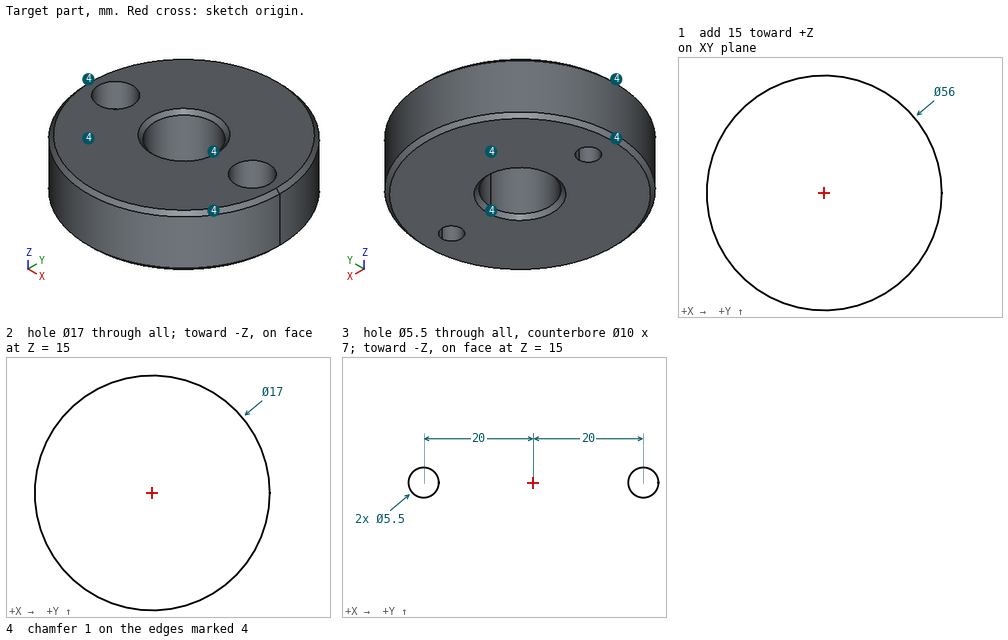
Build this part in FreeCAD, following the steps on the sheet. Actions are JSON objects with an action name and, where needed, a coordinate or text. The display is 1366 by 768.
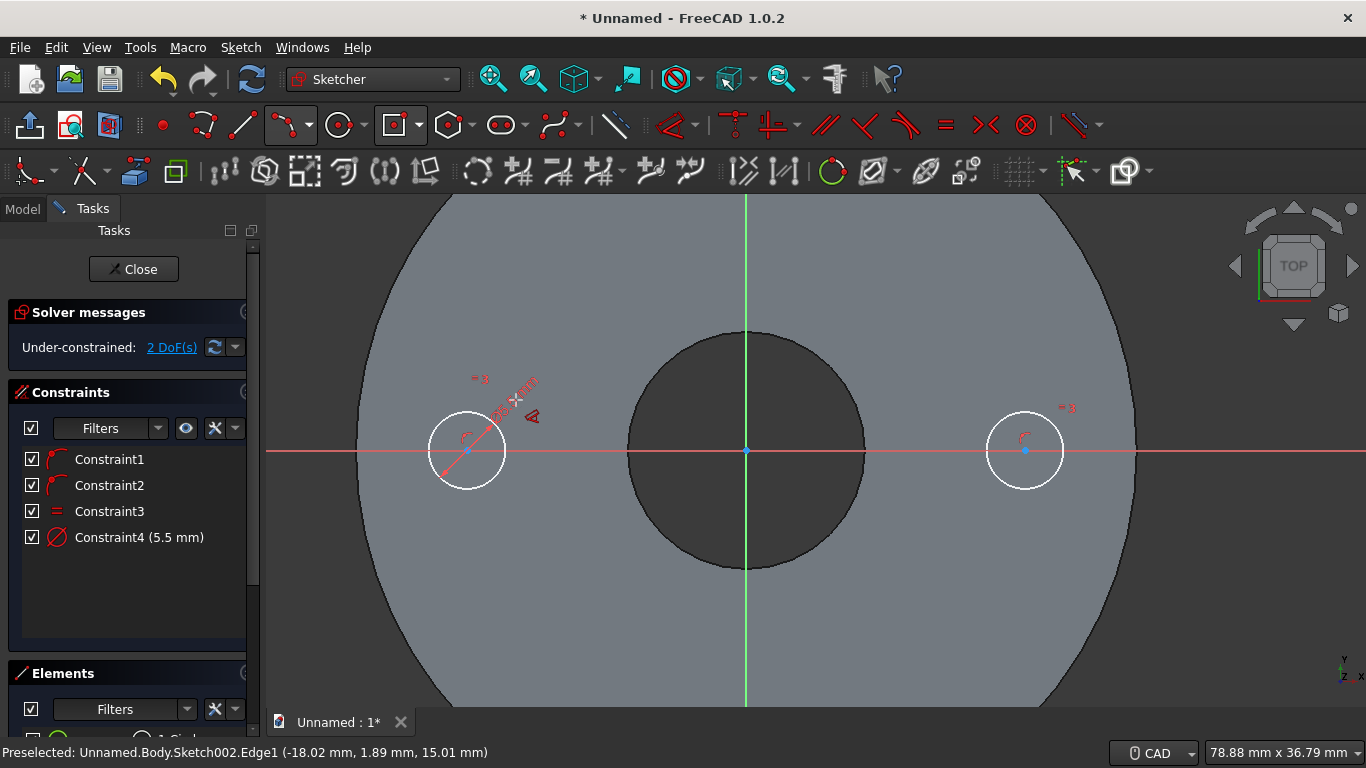
{"action": "left_click", "coordinate": [467, 450]}
{"action": "left_click", "coordinate": [607, 484]}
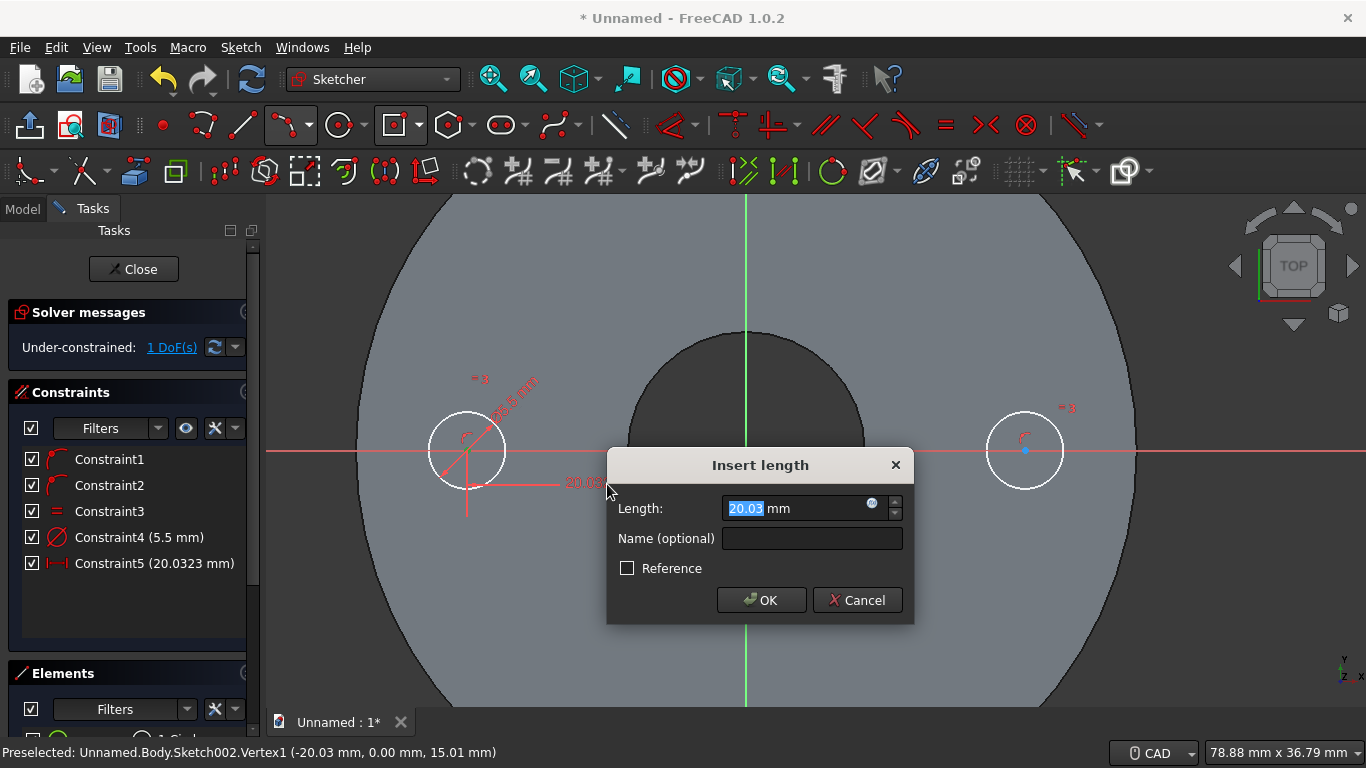
{"action": "type", "text": "20"}
{"action": "key", "text": "Return"}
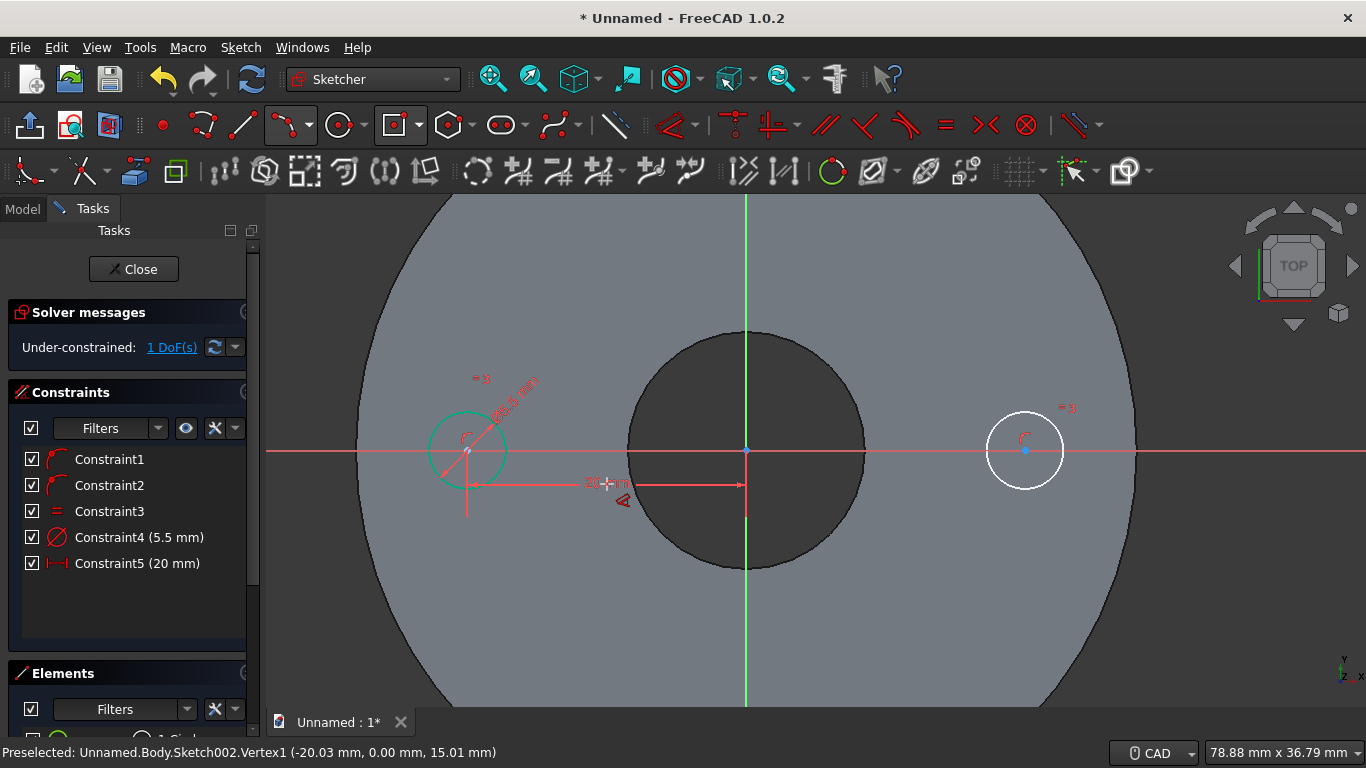
{"action": "left_click", "coordinate": [1025, 450]}
{"action": "left_click", "coordinate": [886, 484]}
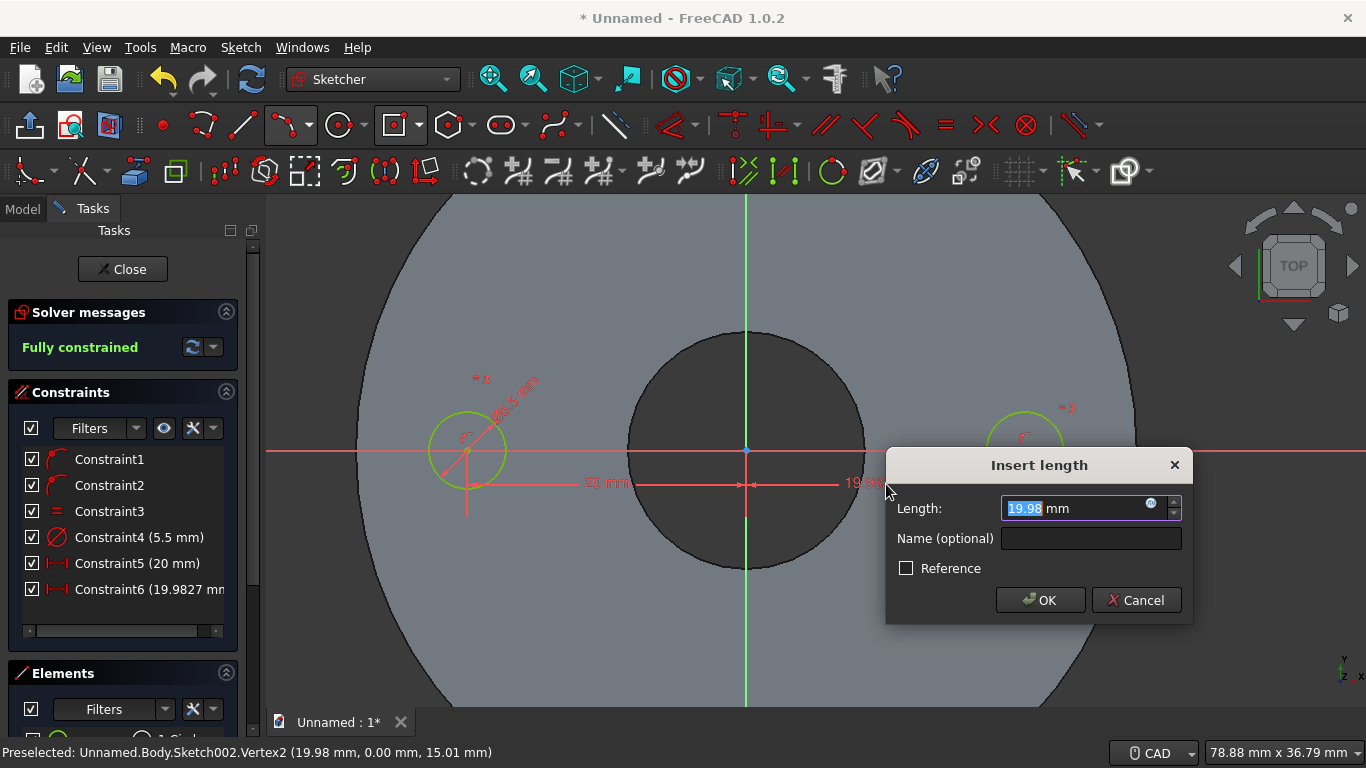
{"action": "type", "text": "20"}
{"action": "key", "text": "Return"}
{"action": "key", "text": "Escape"}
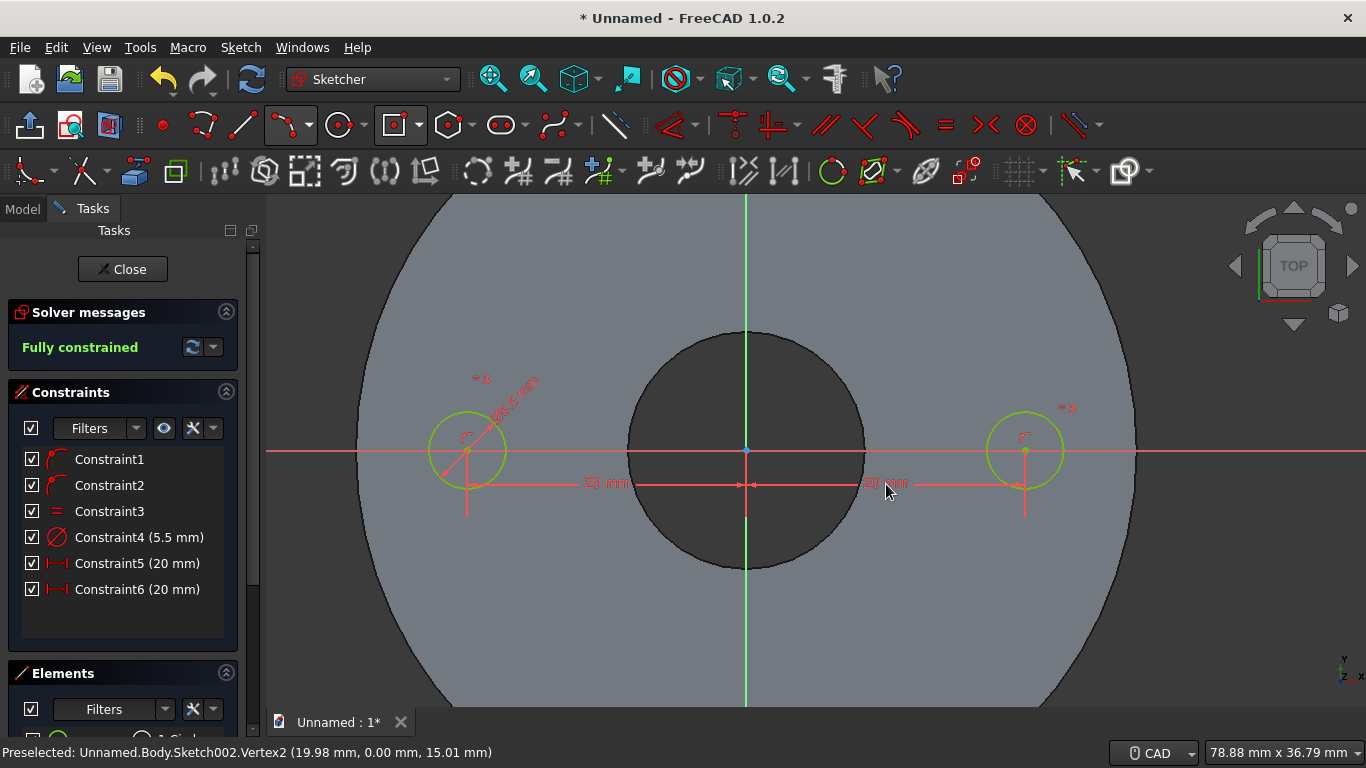
{"action": "left_click", "coordinate": [123, 269]}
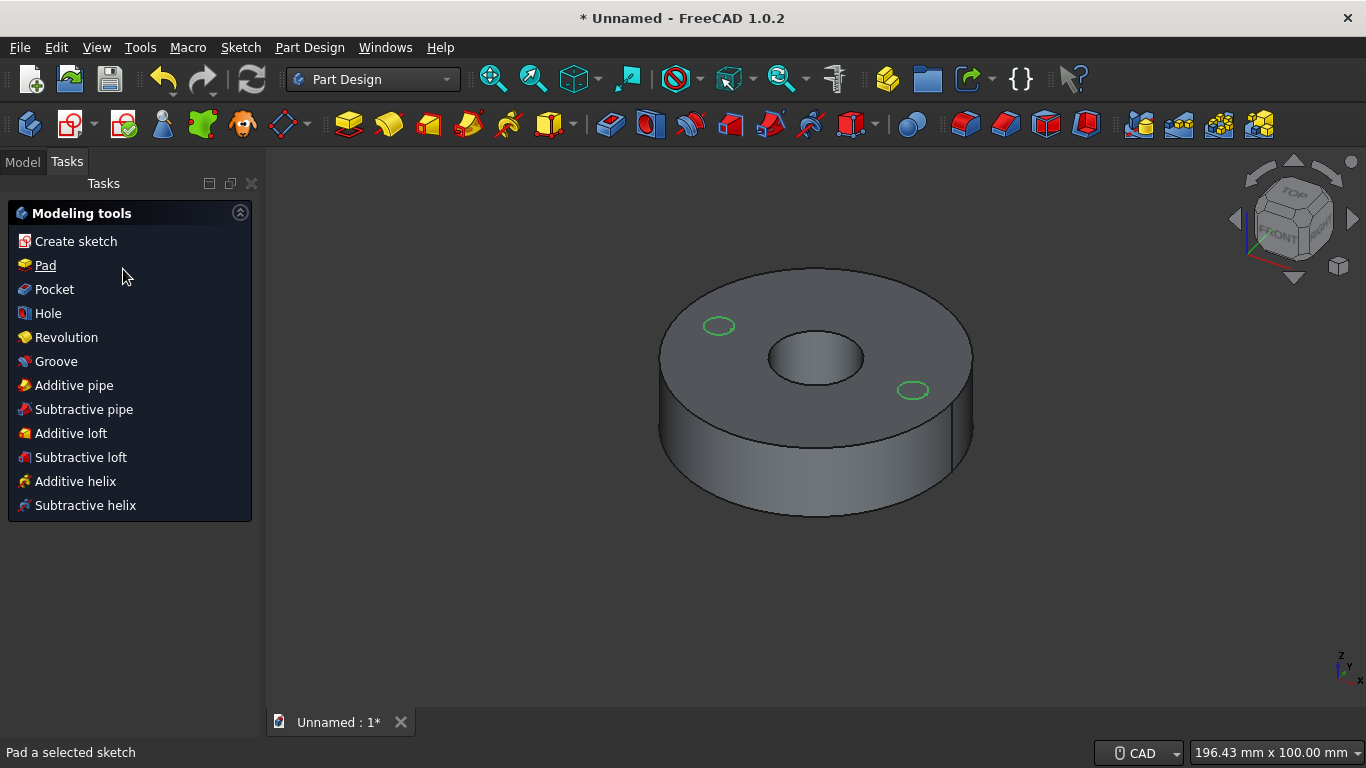
{"action": "left_click", "coordinate": [652, 124]}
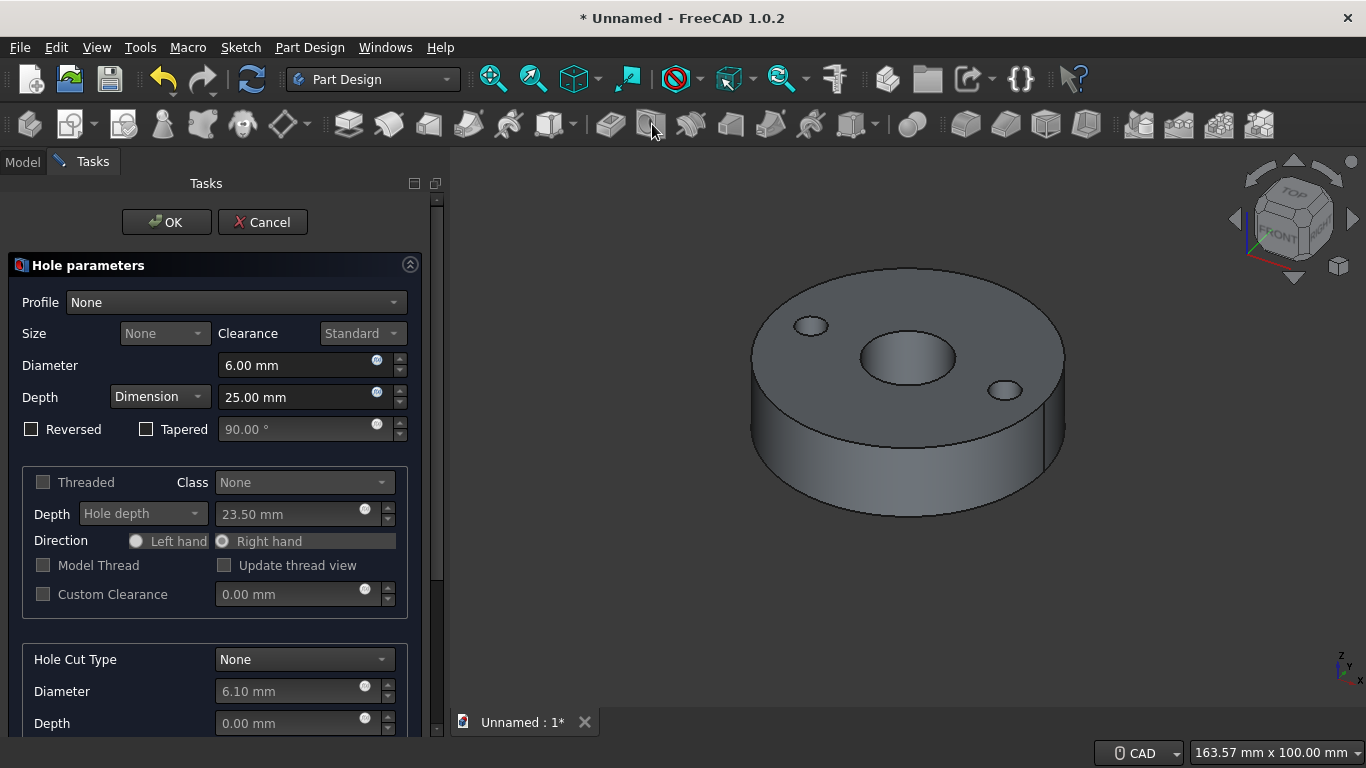
{"action": "triple_click", "coordinate": [305, 365]}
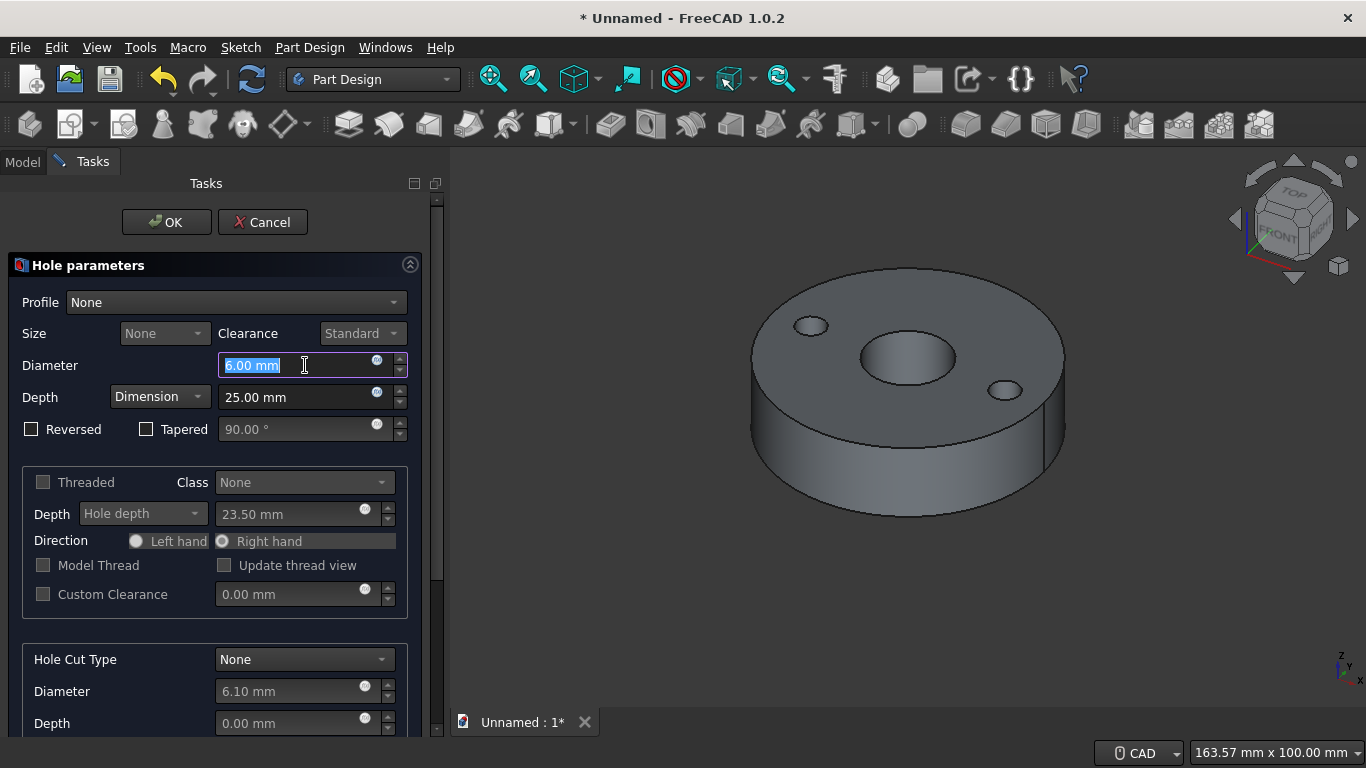
{"action": "type", "text": "5.5"}
{"action": "key", "text": "Tab"}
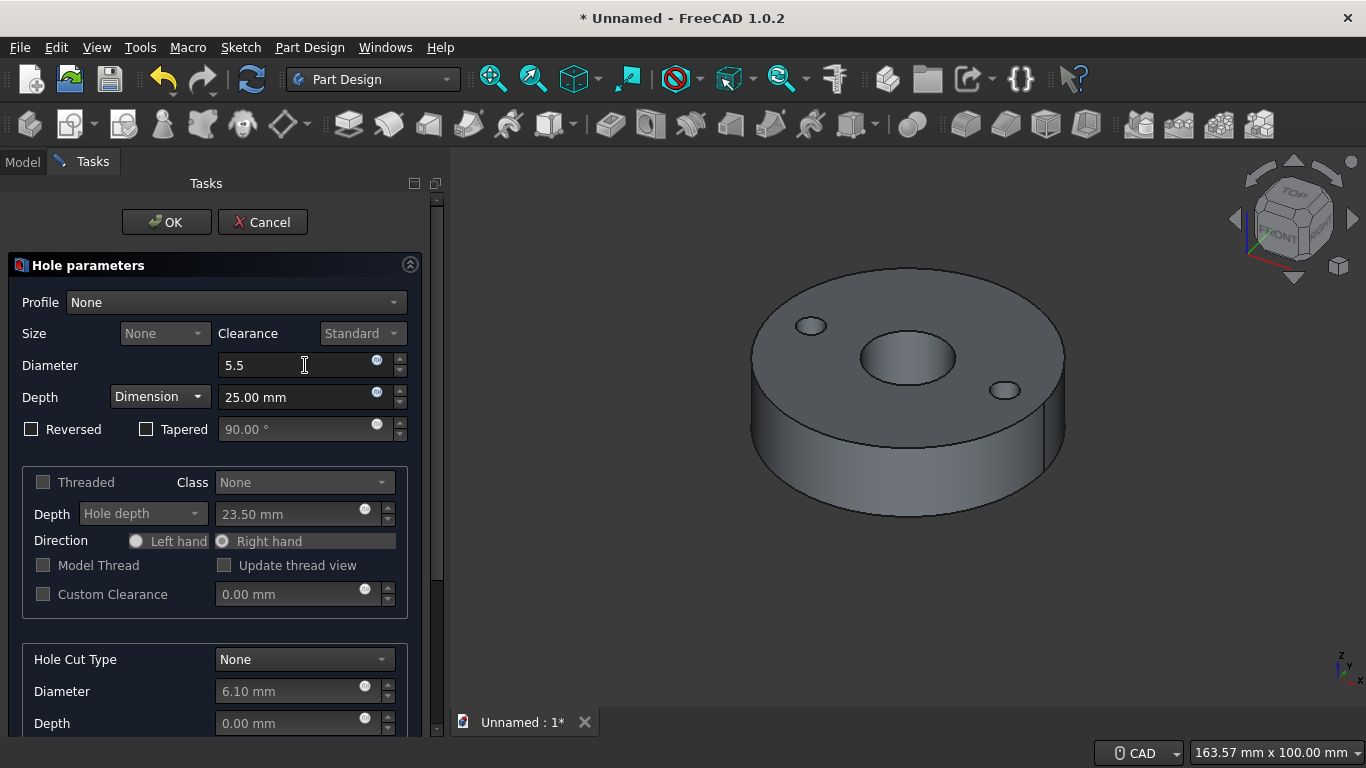
{"action": "left_click", "coordinate": [161, 396]}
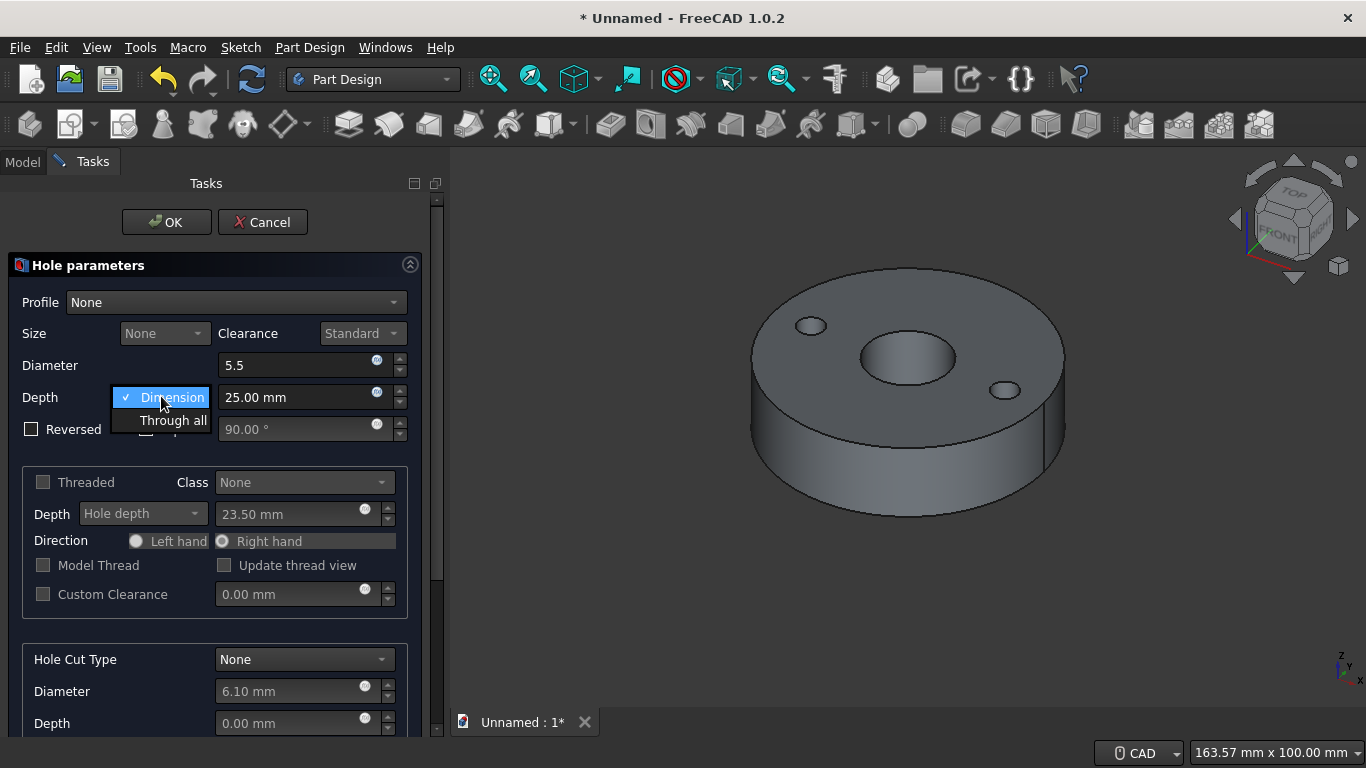
{"action": "left_click", "coordinate": [160, 420]}